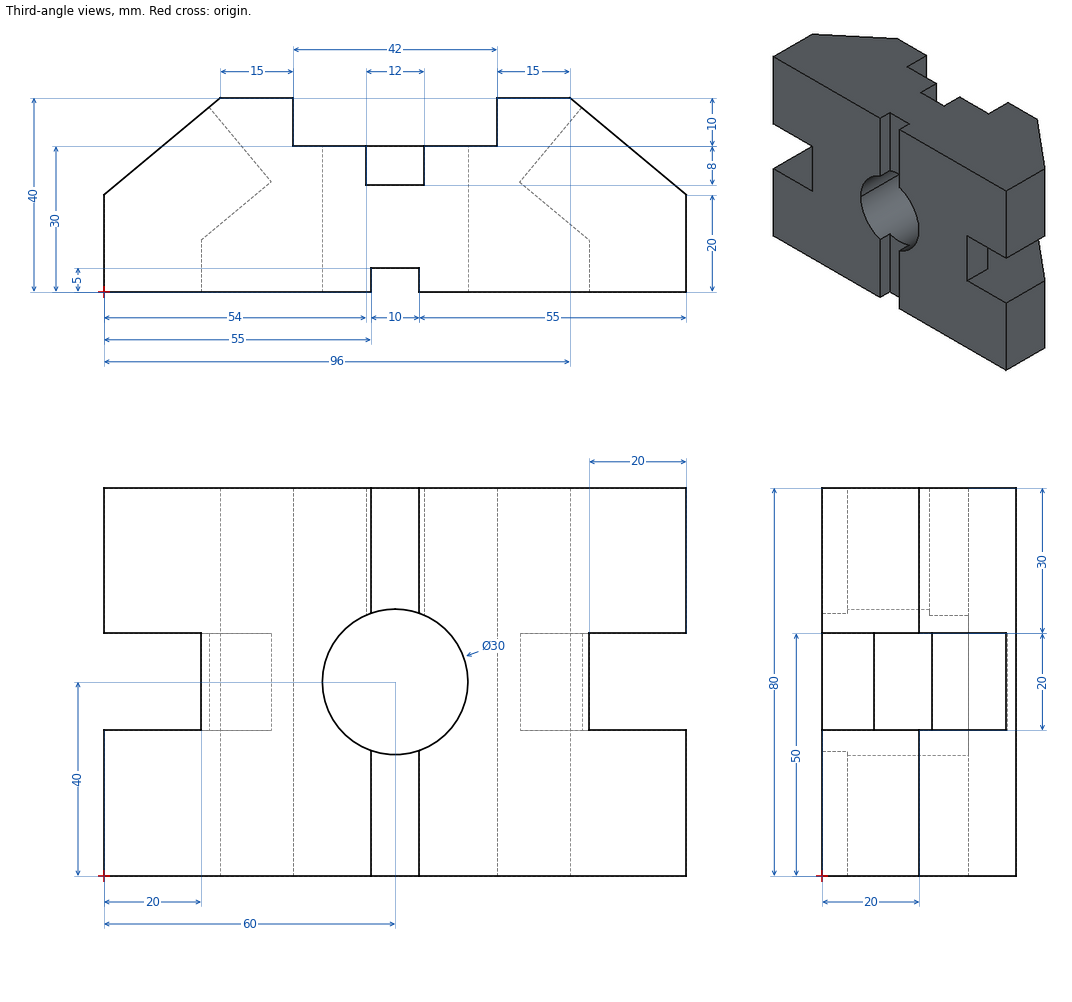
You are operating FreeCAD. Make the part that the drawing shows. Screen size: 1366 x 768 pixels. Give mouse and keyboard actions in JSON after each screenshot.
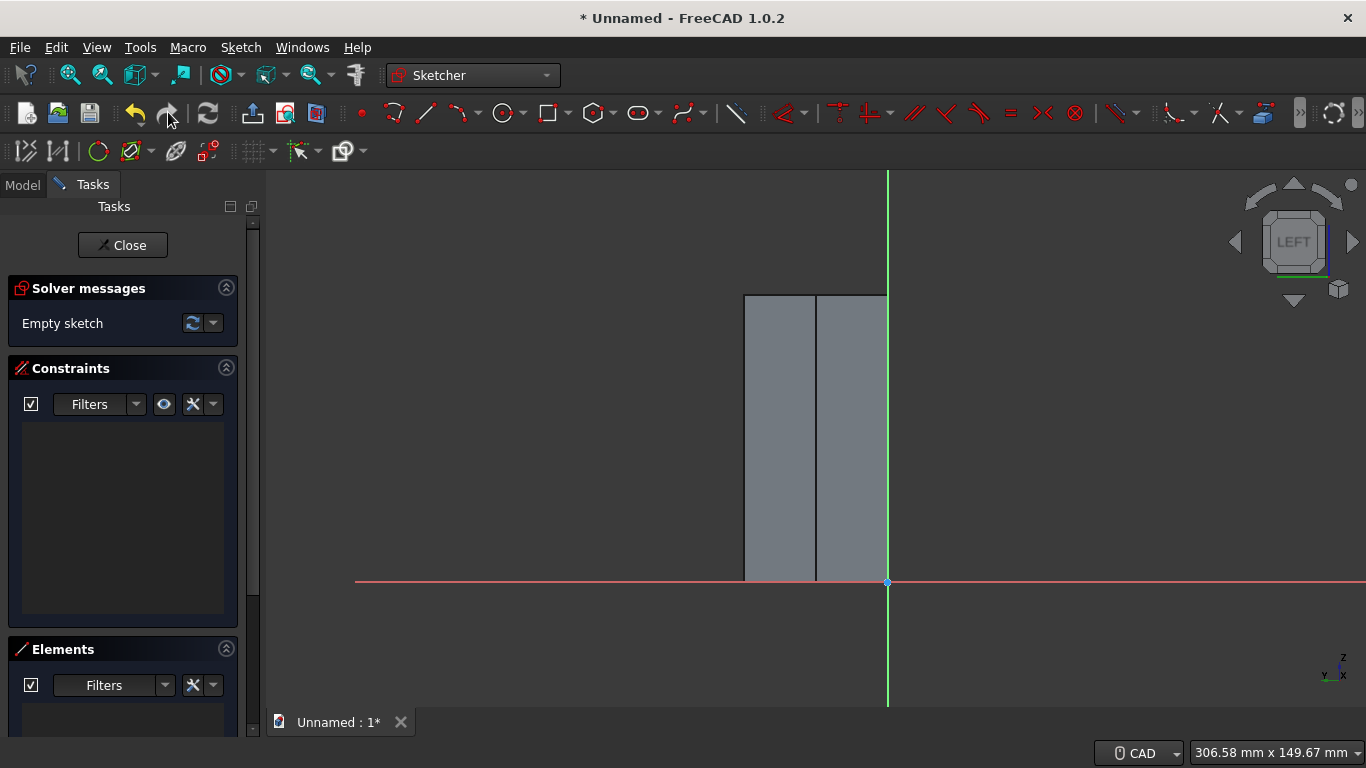
{"action": "scroll", "coordinate": [878, 439], "scroll_direction": "up", "scroll_amount": 8}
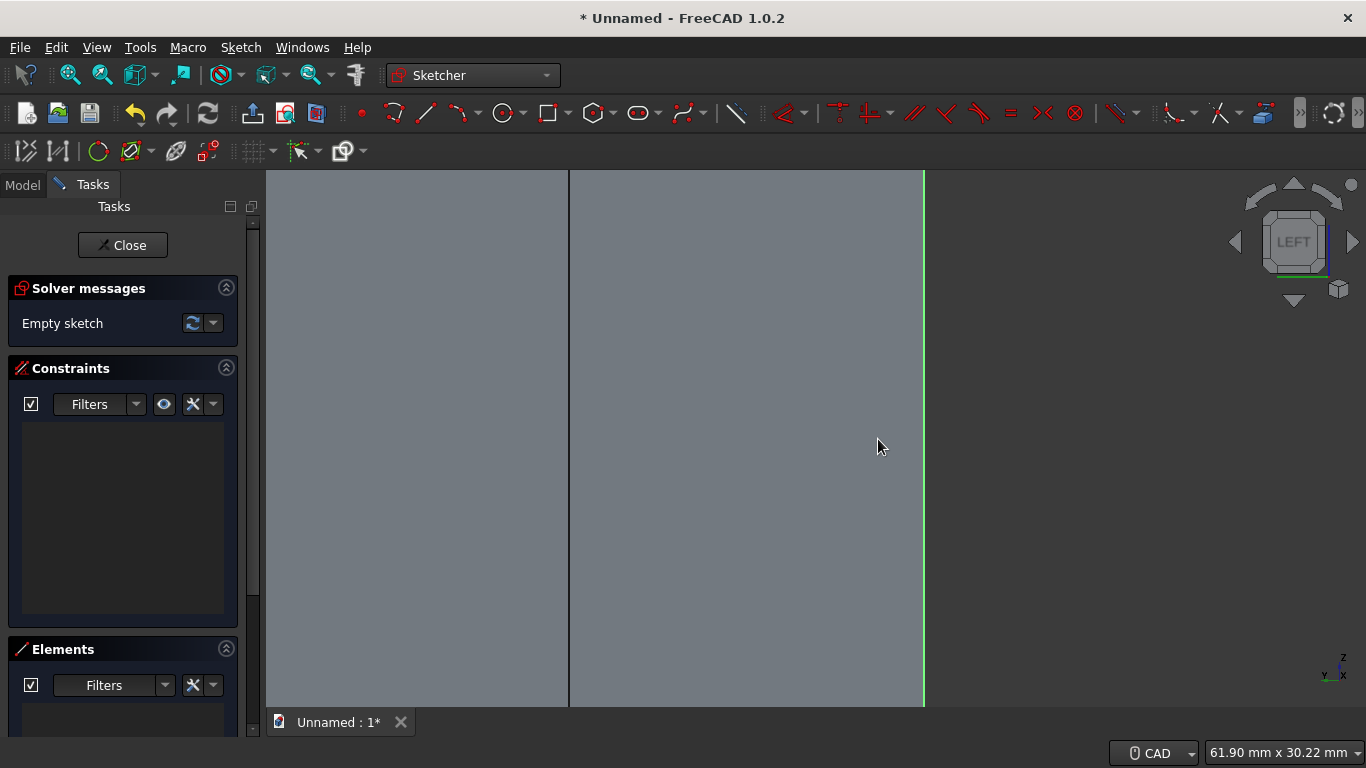
{"action": "key", "text": "g r"}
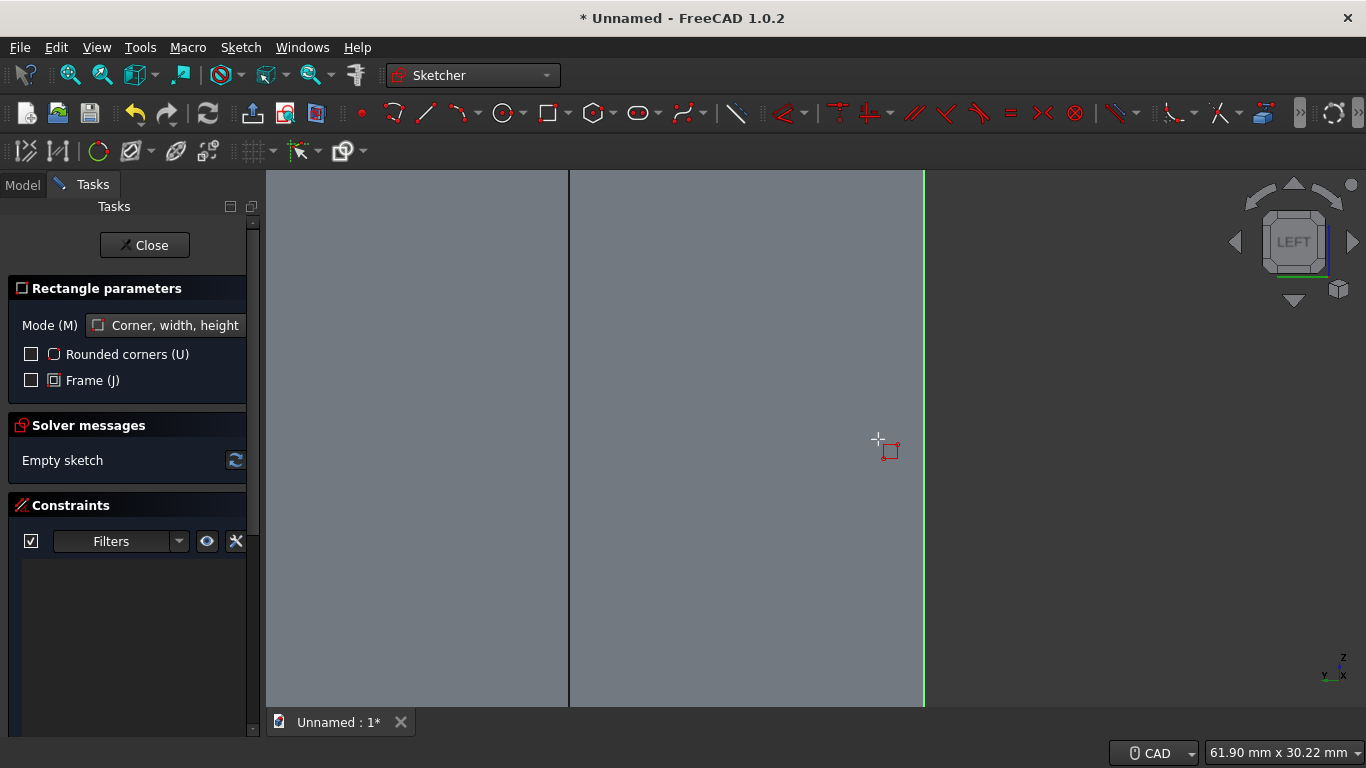
{"action": "left_click", "coordinate": [569, 257]}
{"action": "left_click", "coordinate": [924, 612]}
{"action": "key", "text": "Escape"}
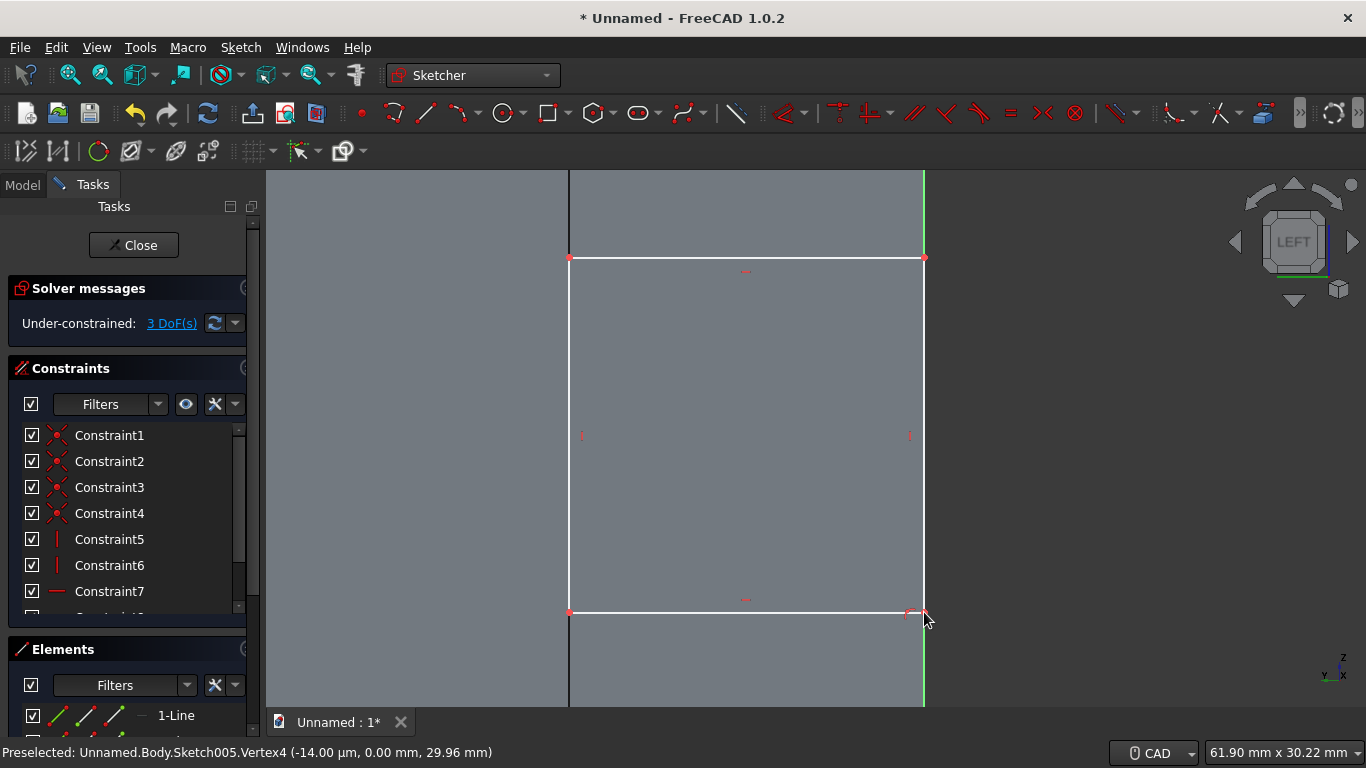
{"action": "key", "text": "d"}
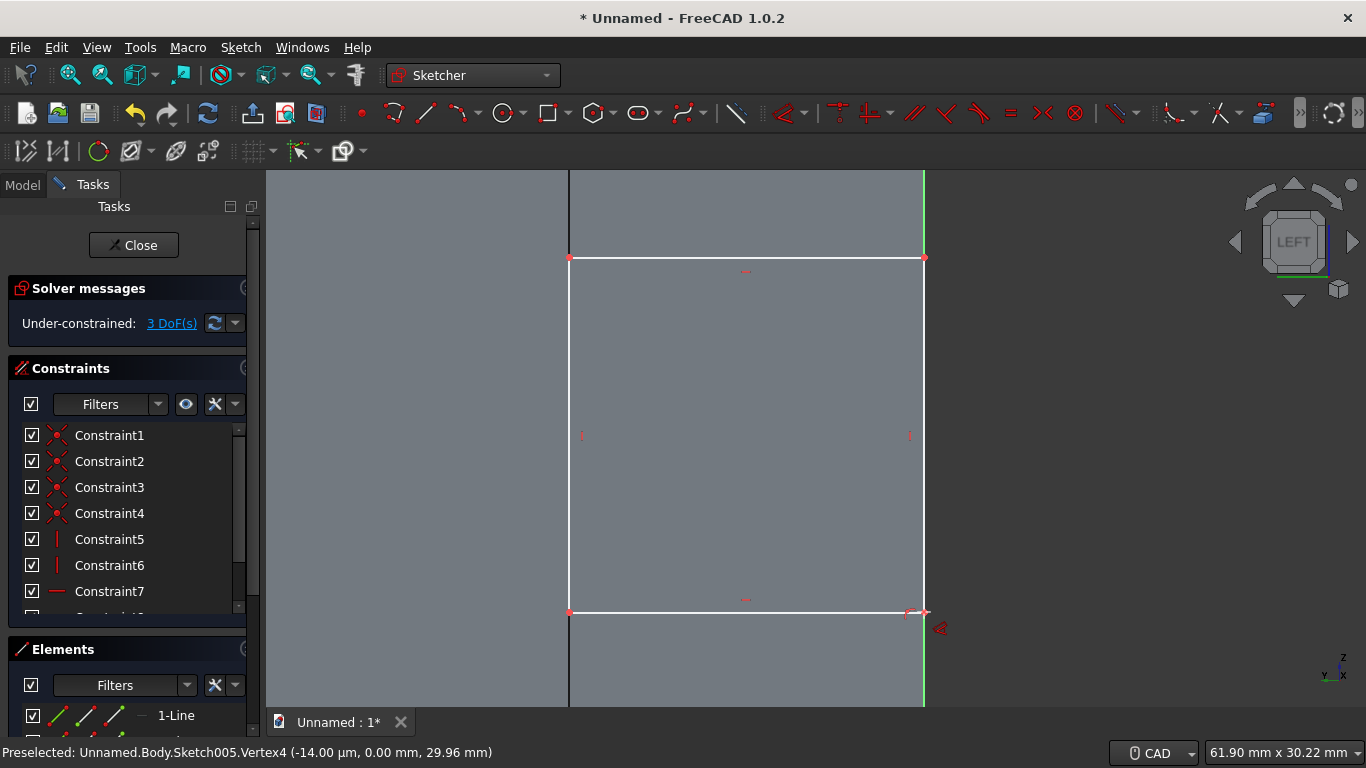
{"action": "left_click", "coordinate": [569, 364]}
{"action": "left_click", "coordinate": [535, 435]}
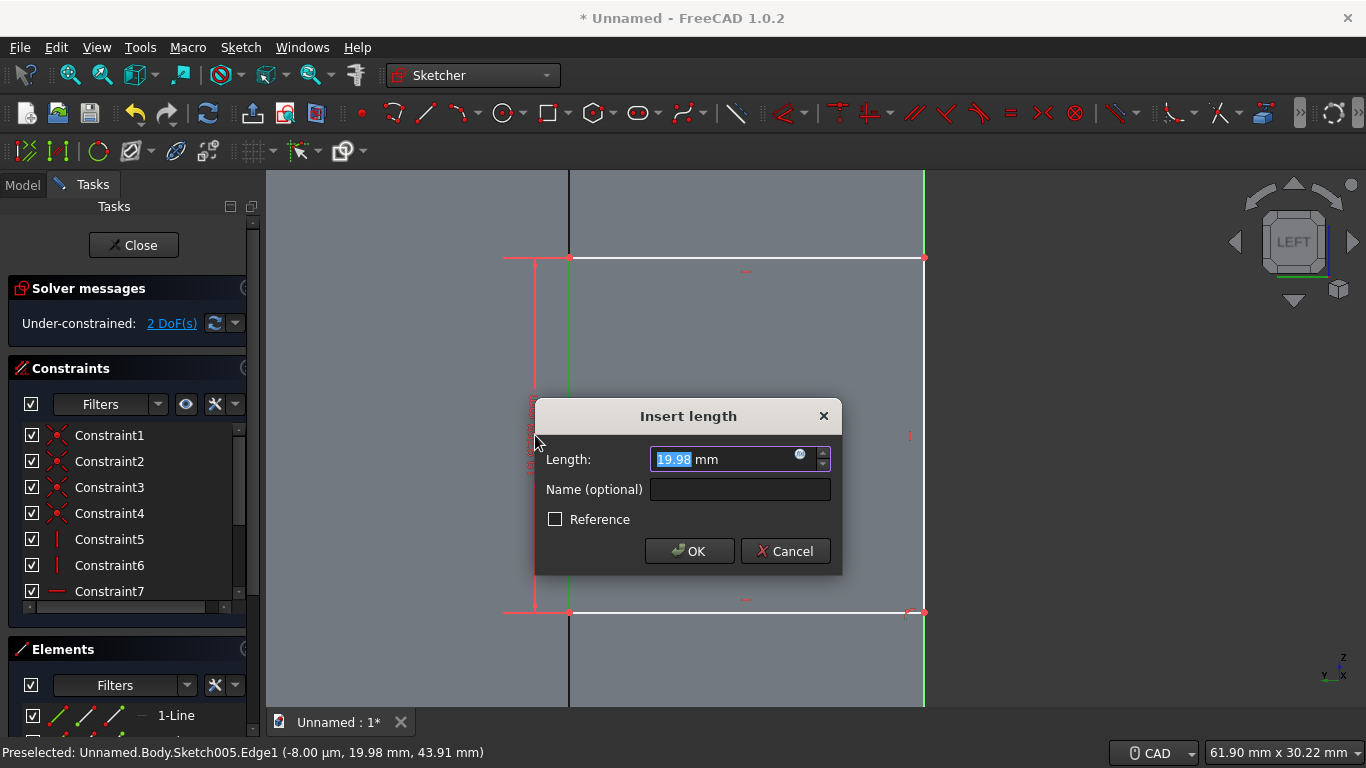
{"action": "type", "text": "20"}
{"action": "key", "text": "Return"}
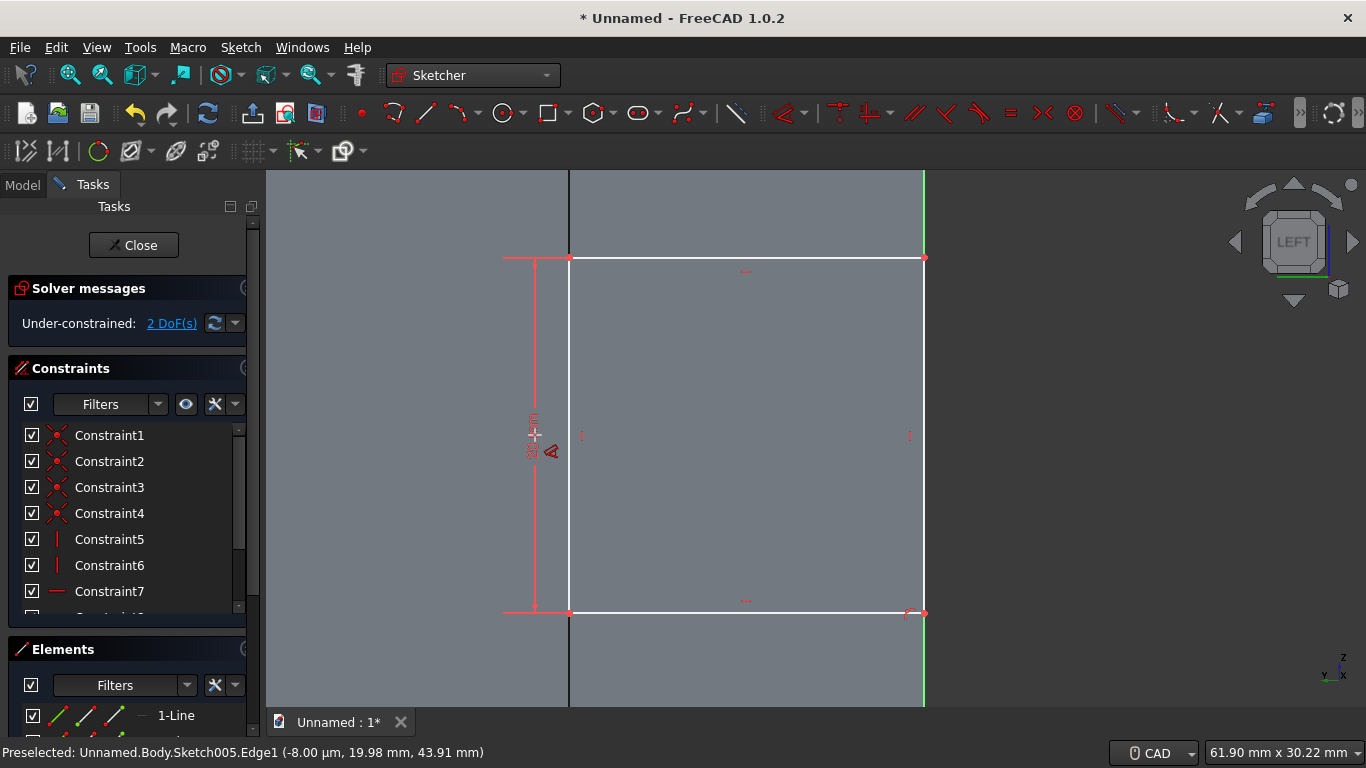
{"action": "left_click", "coordinate": [676, 613]}
{"action": "left_click", "coordinate": [747, 647]}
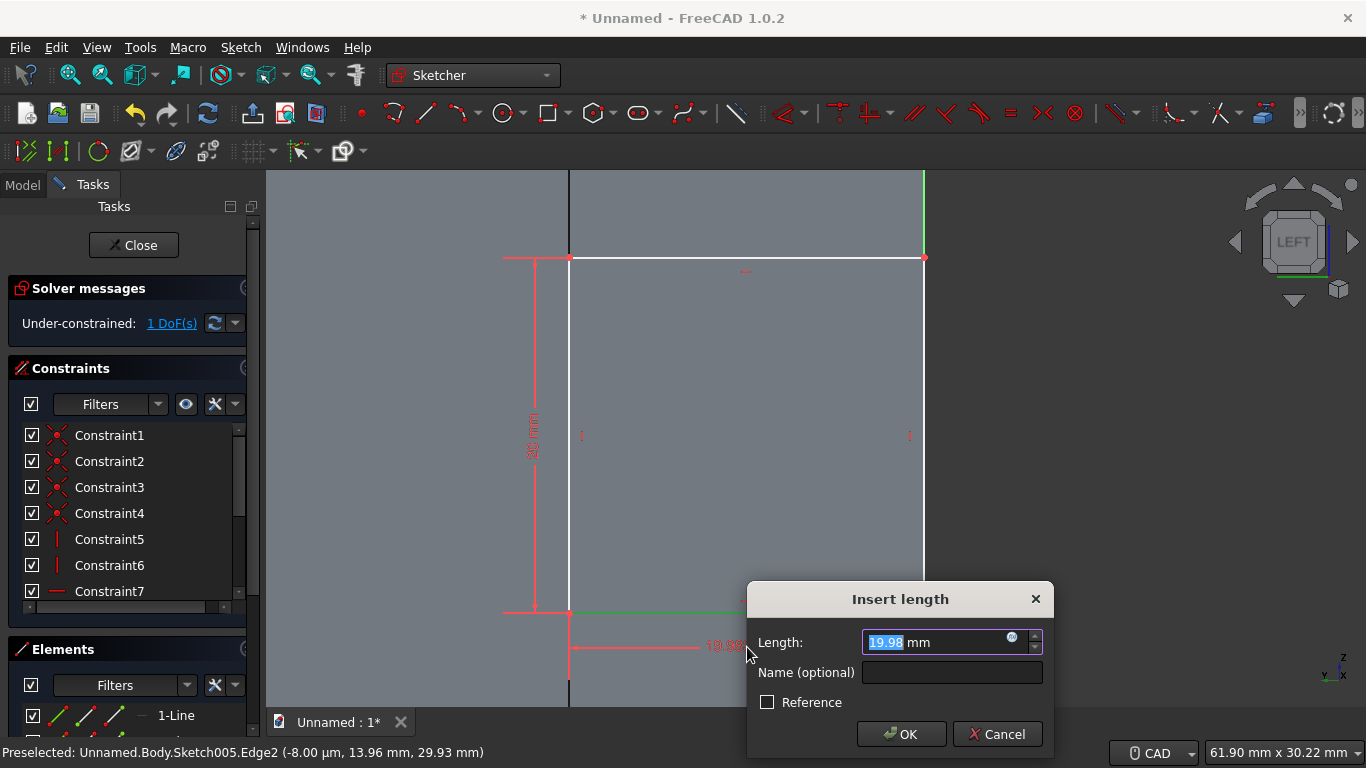
{"action": "type", "text": "20"}
{"action": "key", "text": "Return"}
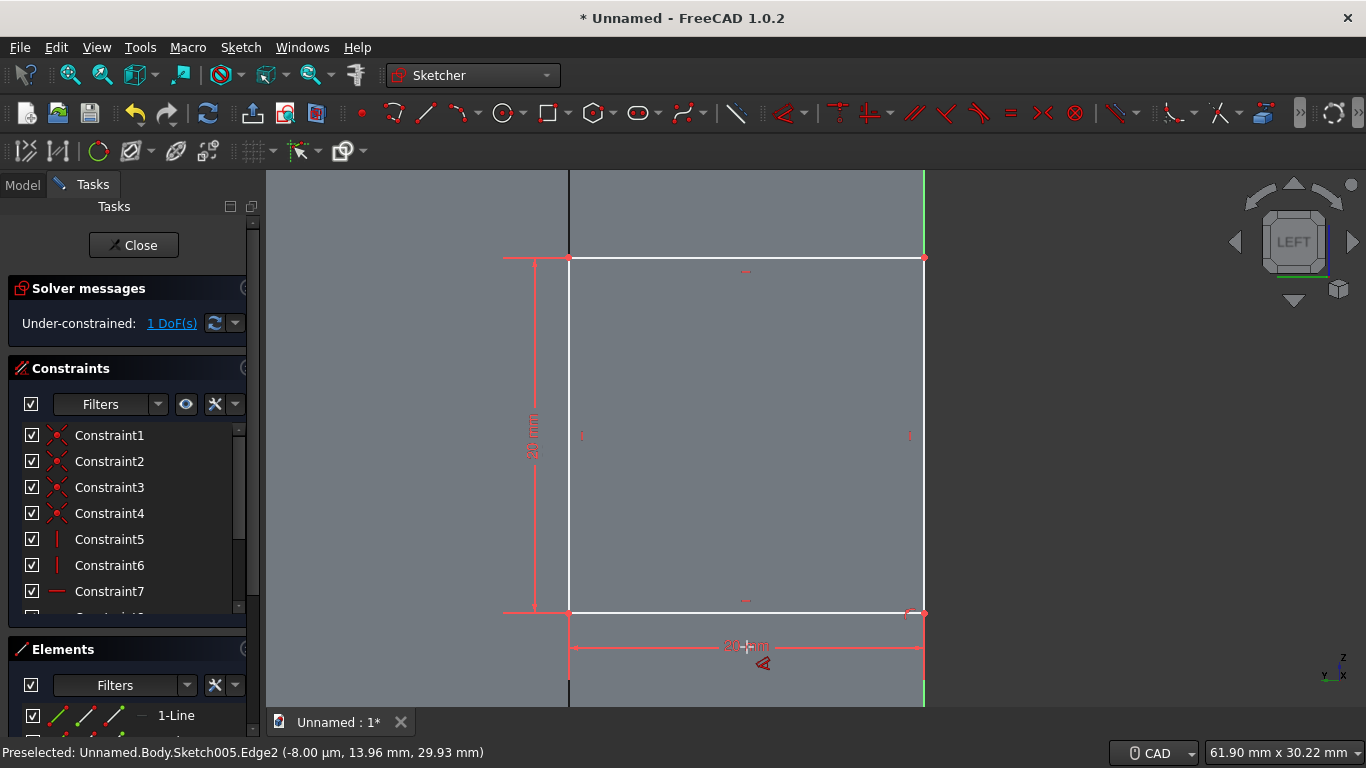
{"action": "left_click", "coordinate": [569, 258]}
{"action": "left_click", "coordinate": [958, 468]}